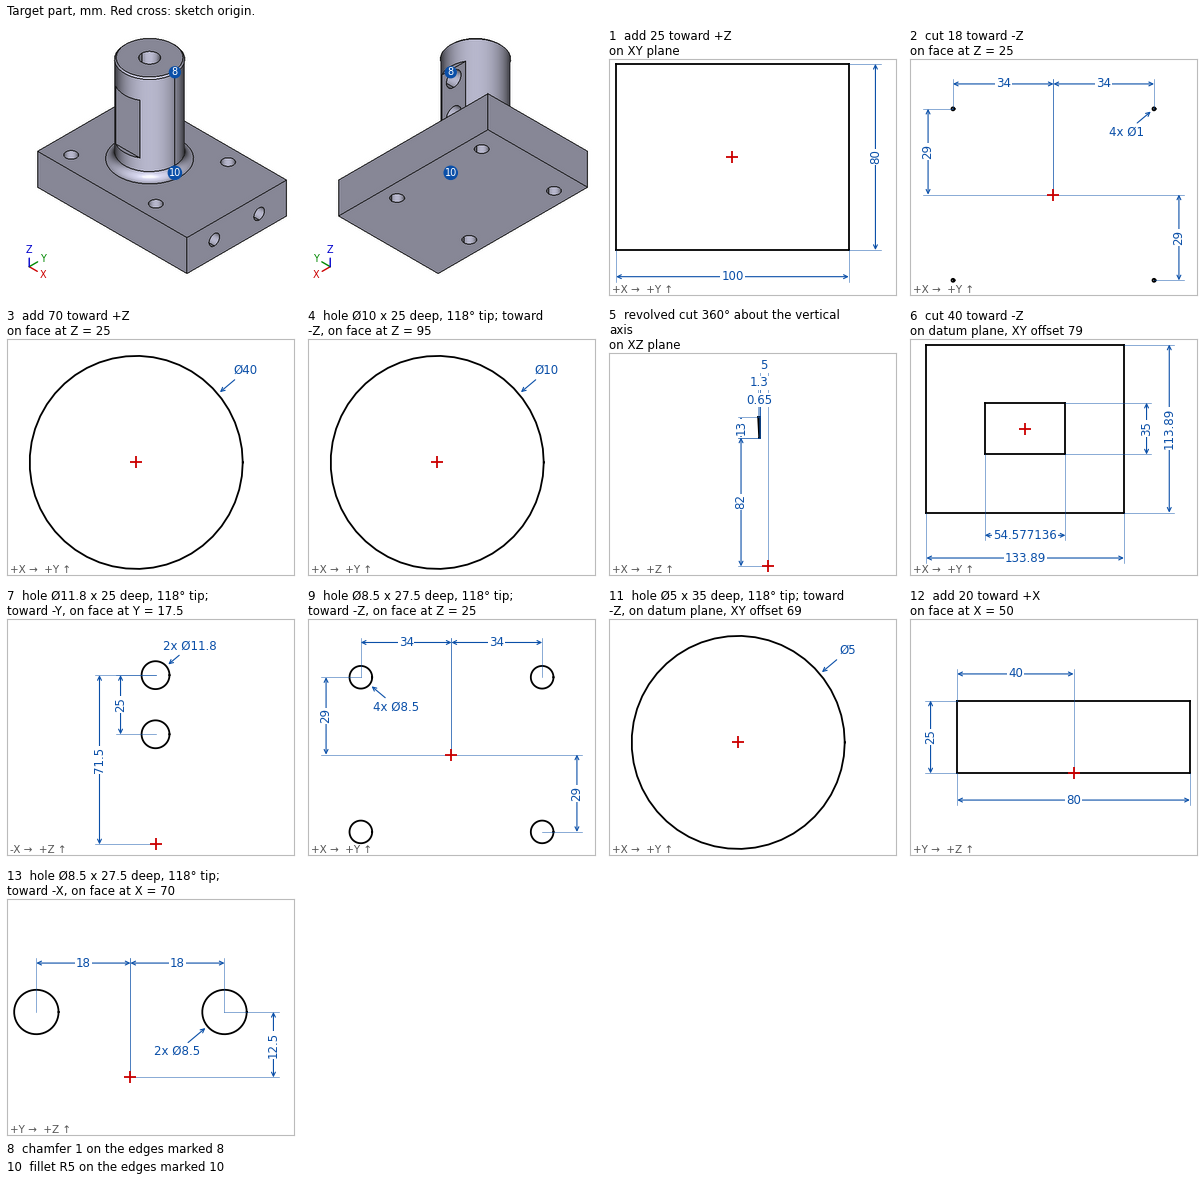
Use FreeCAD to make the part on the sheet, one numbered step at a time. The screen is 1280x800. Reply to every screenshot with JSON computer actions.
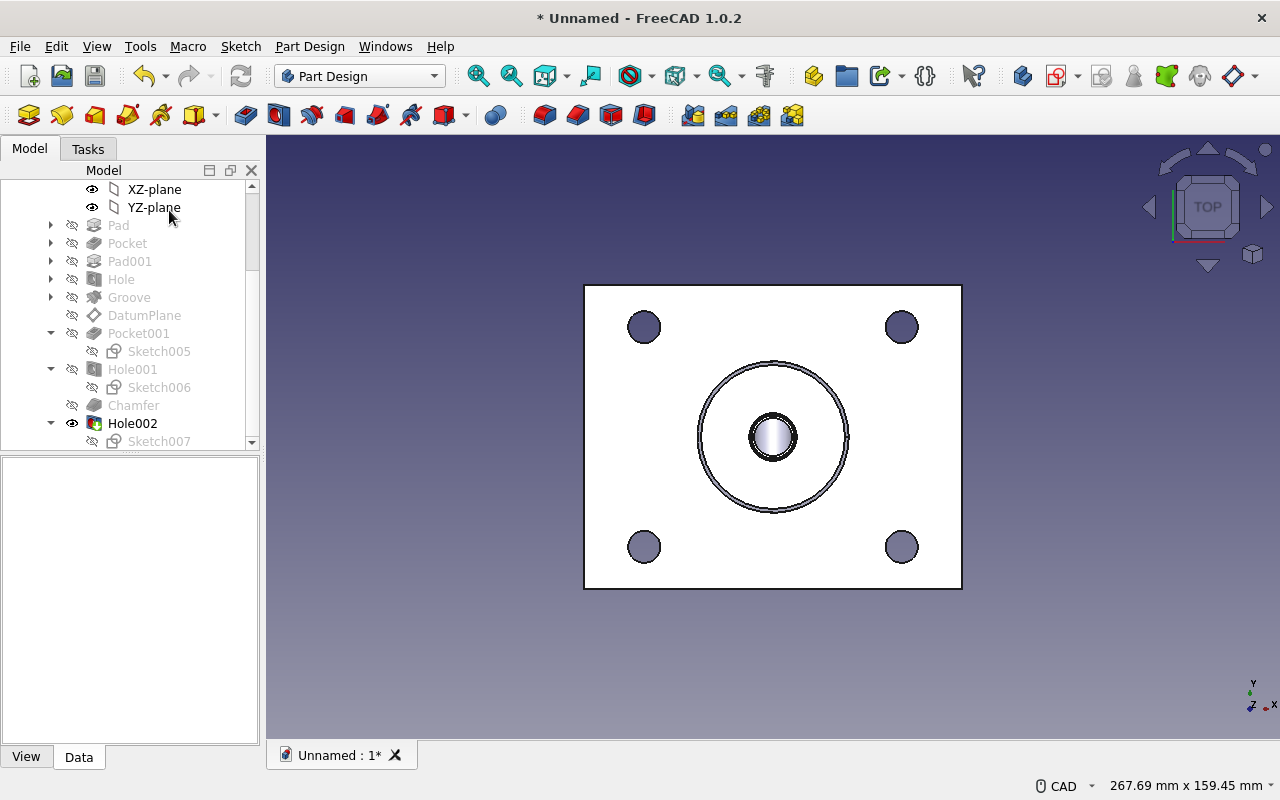
{"action": "key", "text": "0"}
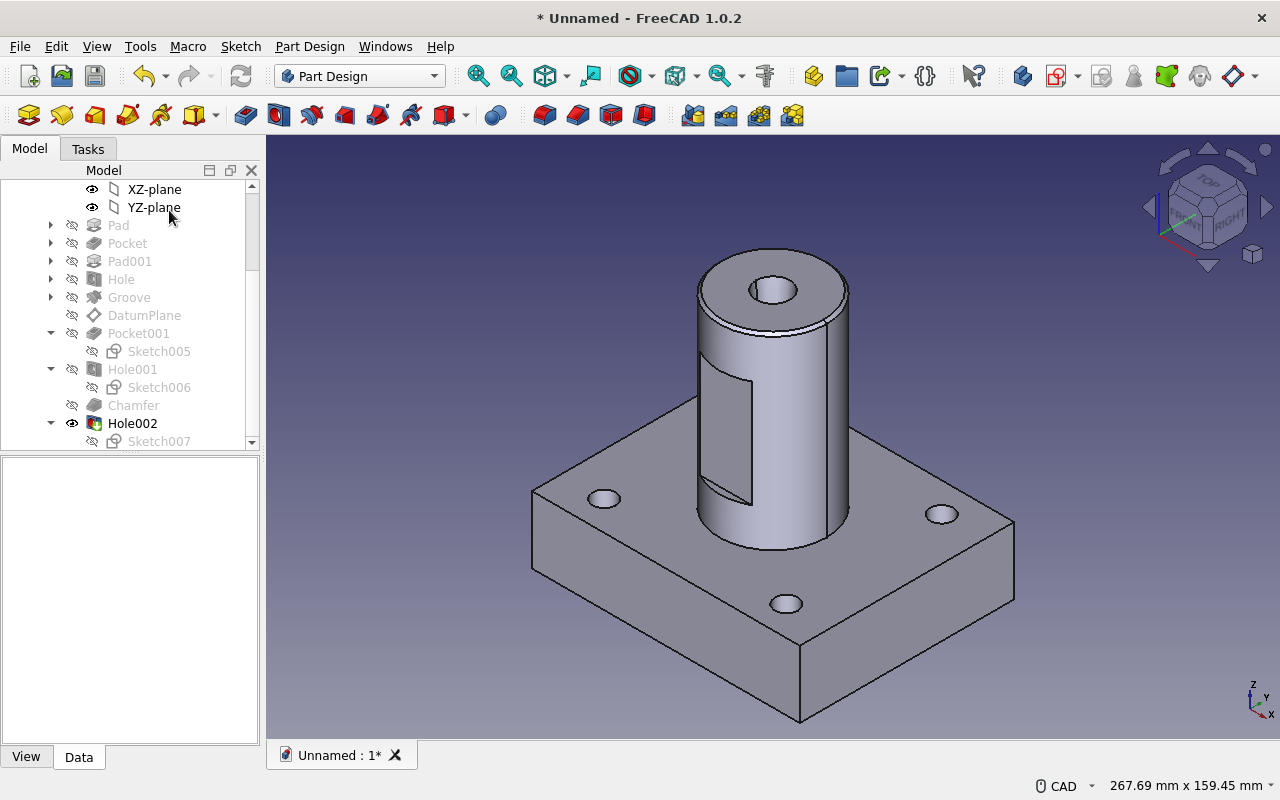
{"action": "key", "text": "1"}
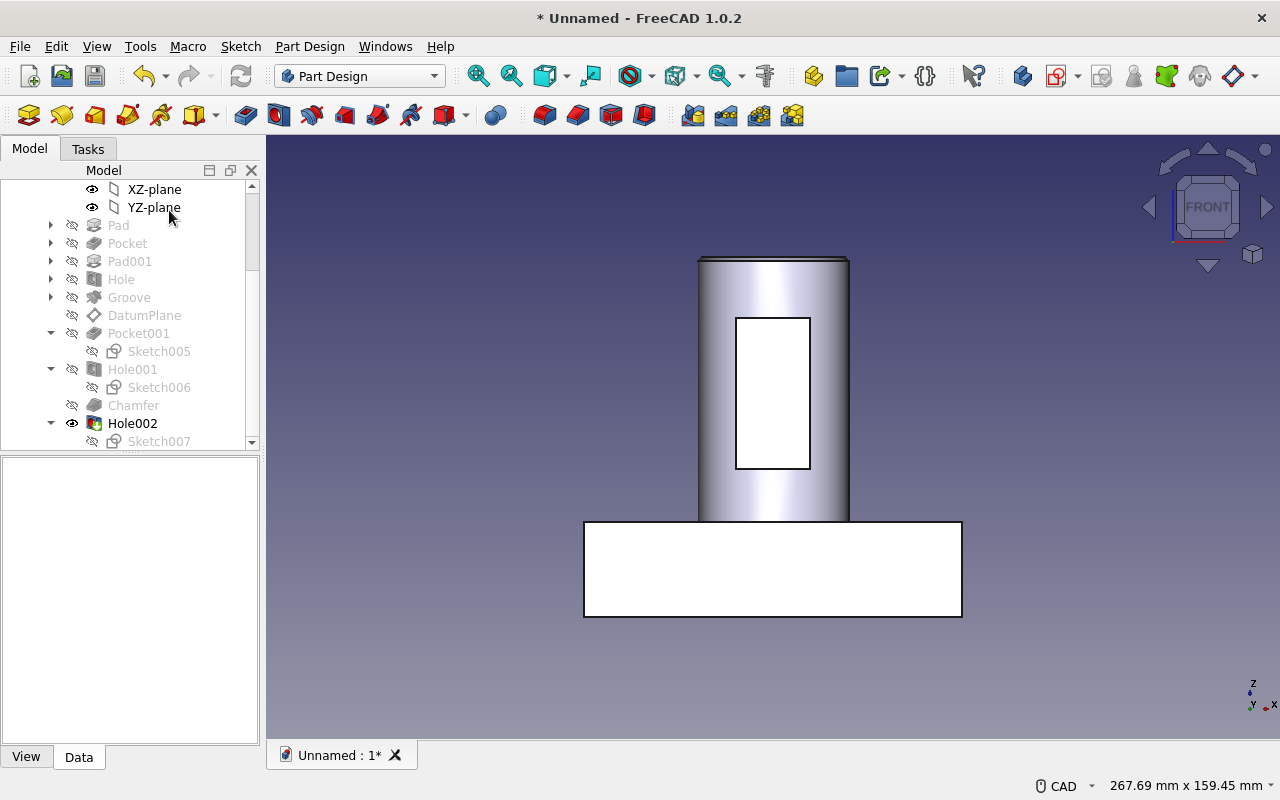
{"action": "key", "text": "3"}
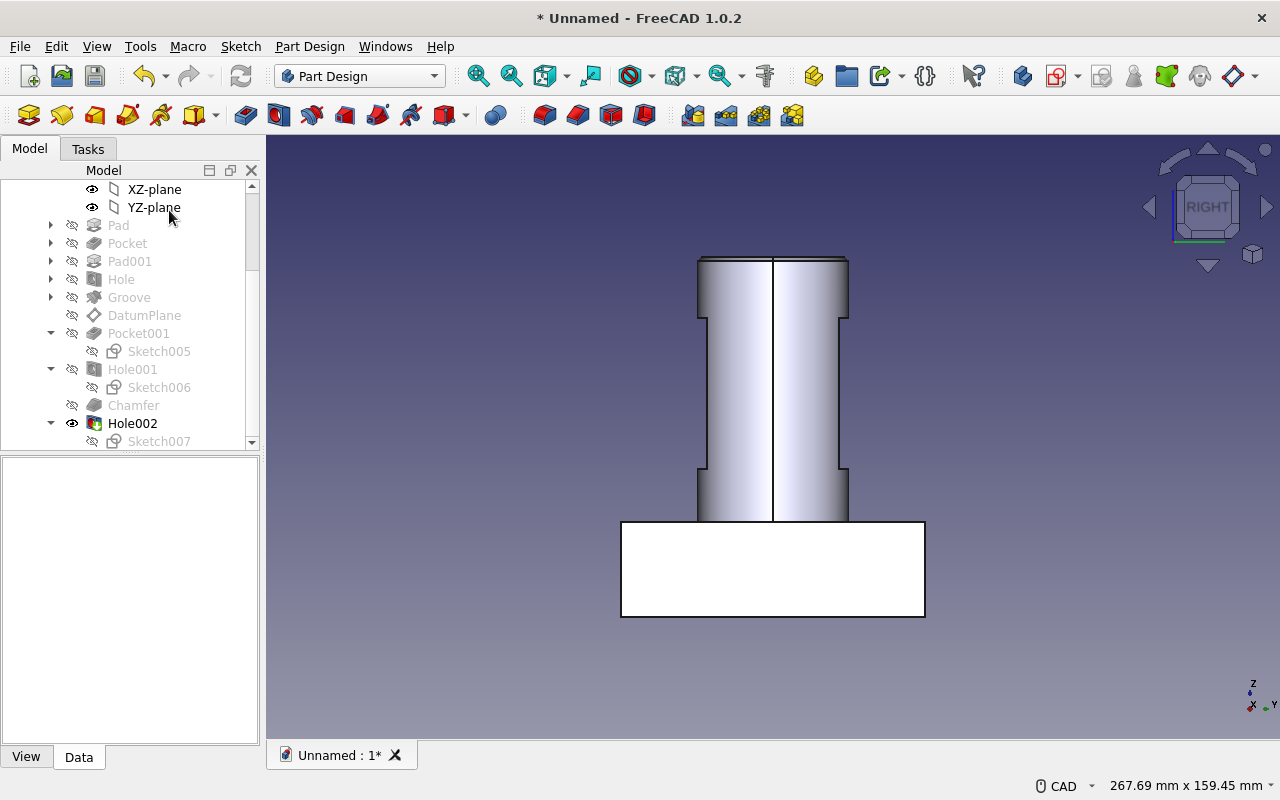
{"action": "key", "text": "5"}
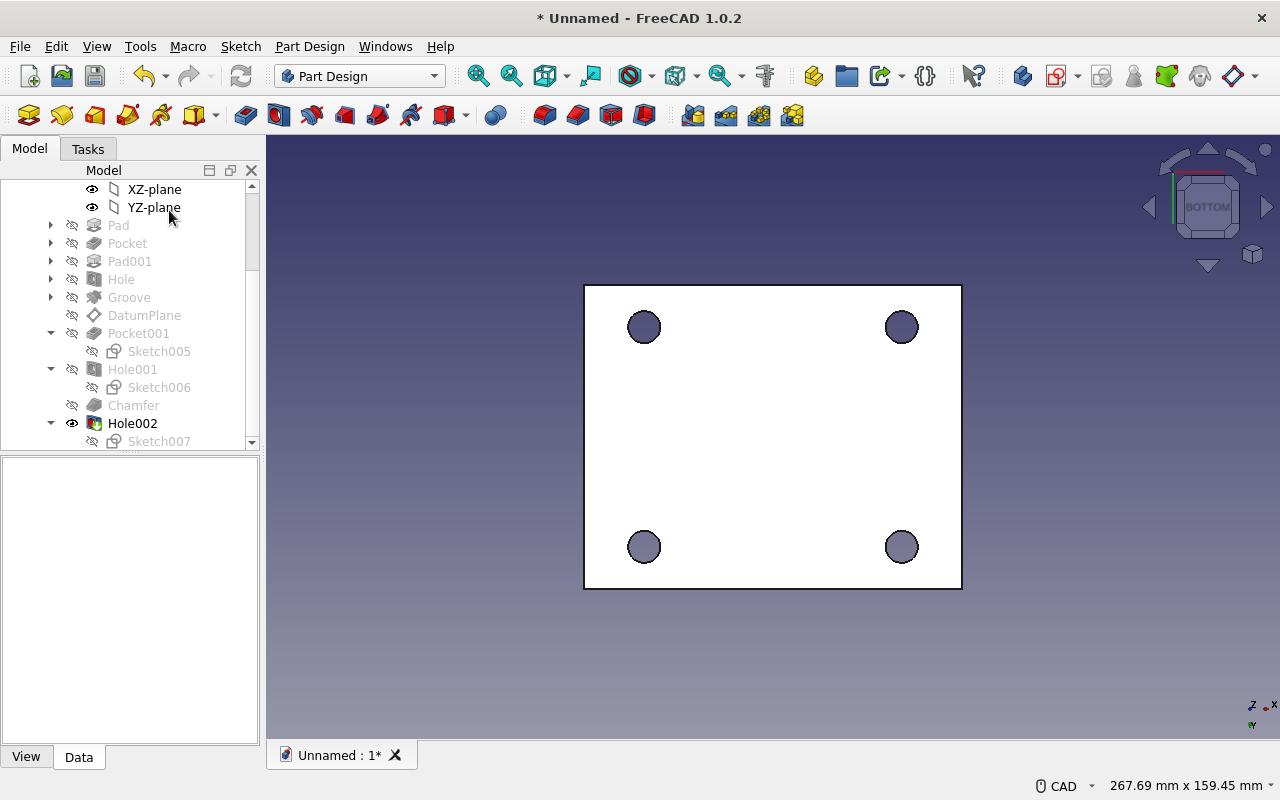
{"action": "key", "text": "4"}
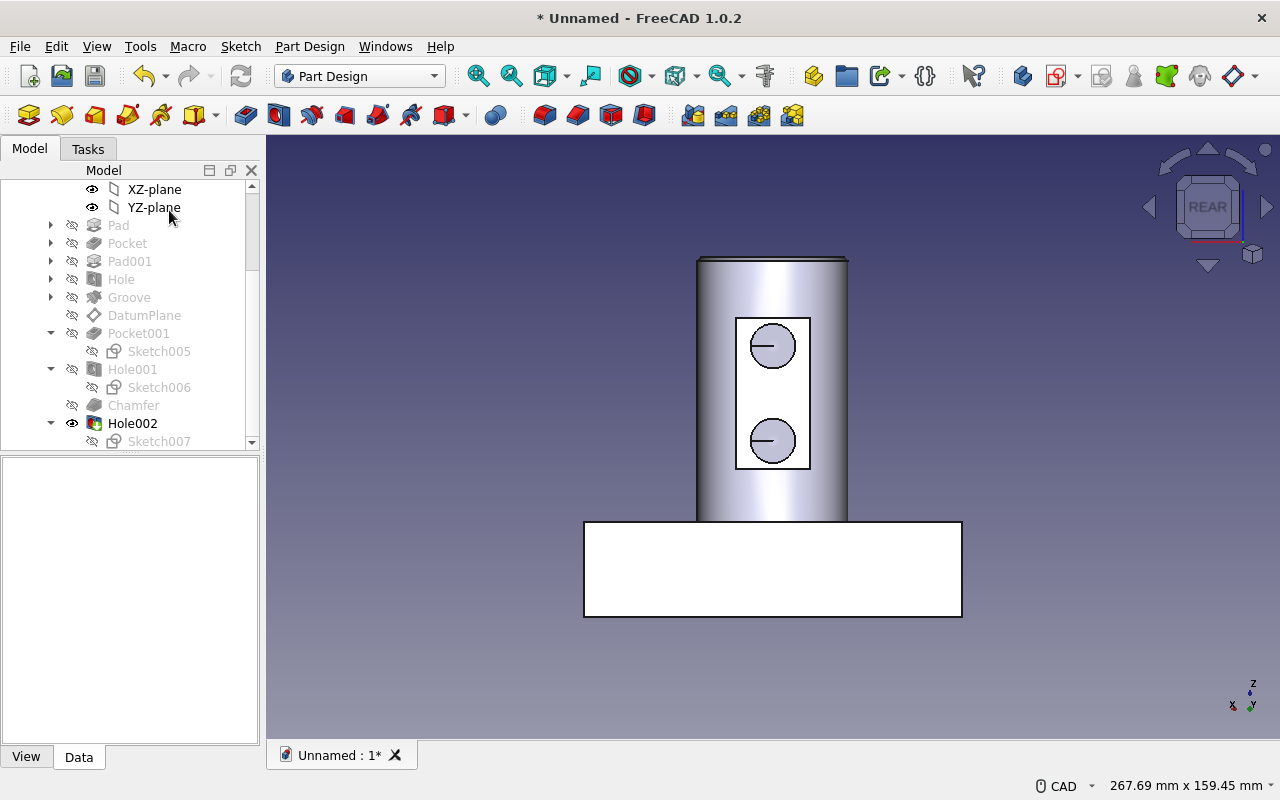
{"action": "key", "text": "6"}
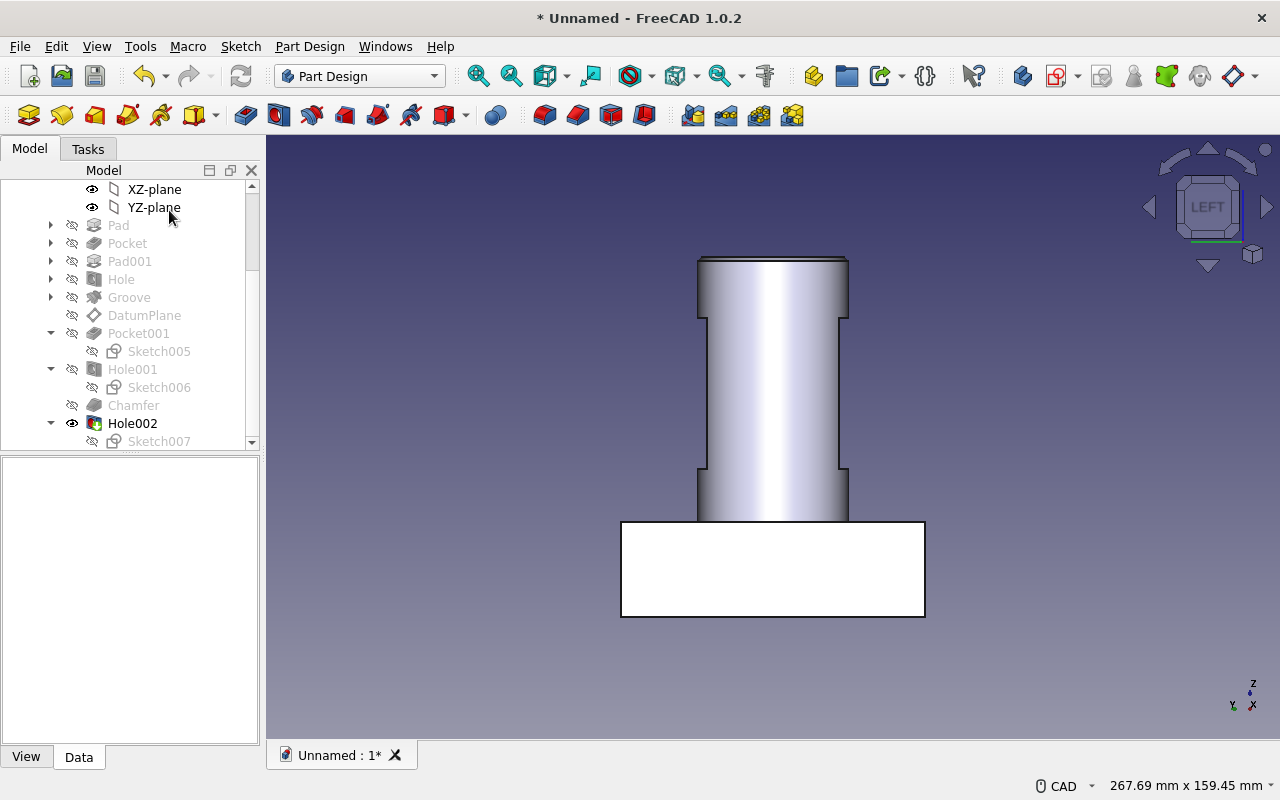
{"action": "key", "text": "v 3"}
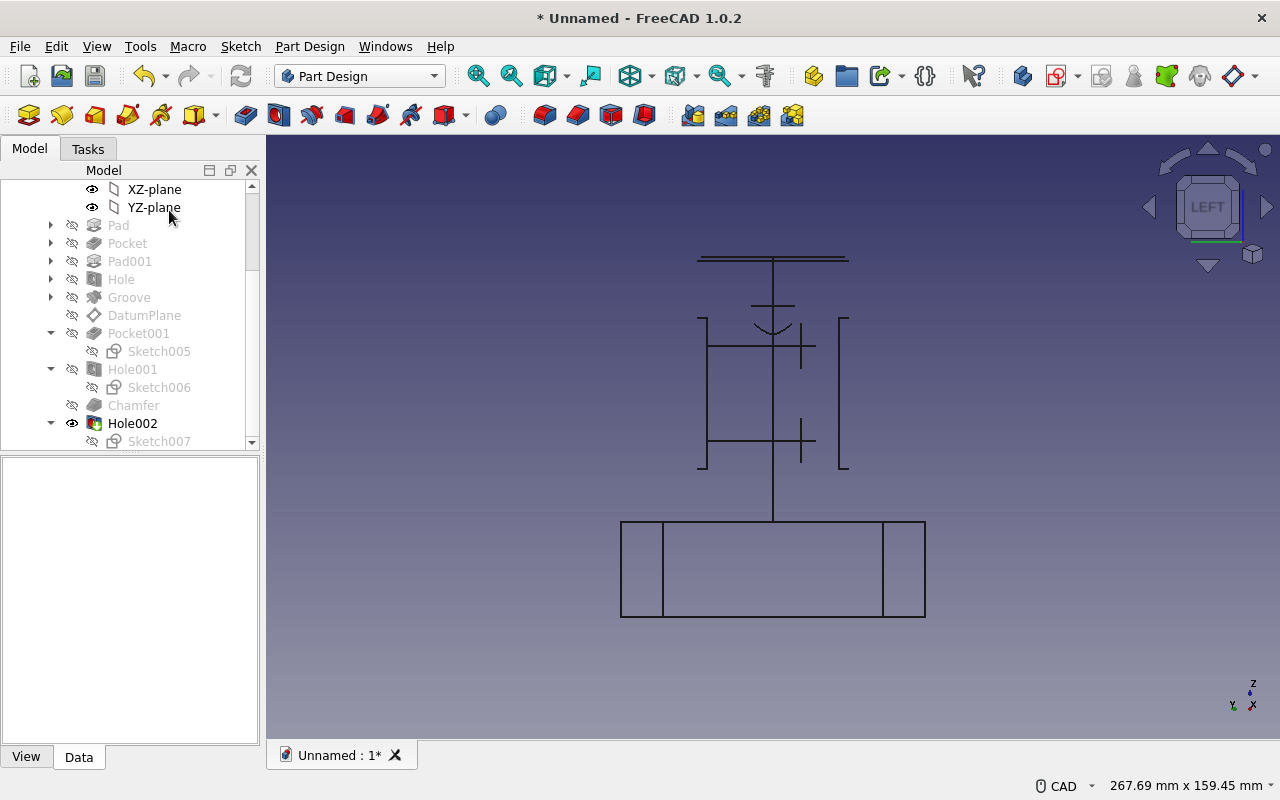
{"action": "key", "text": "0"}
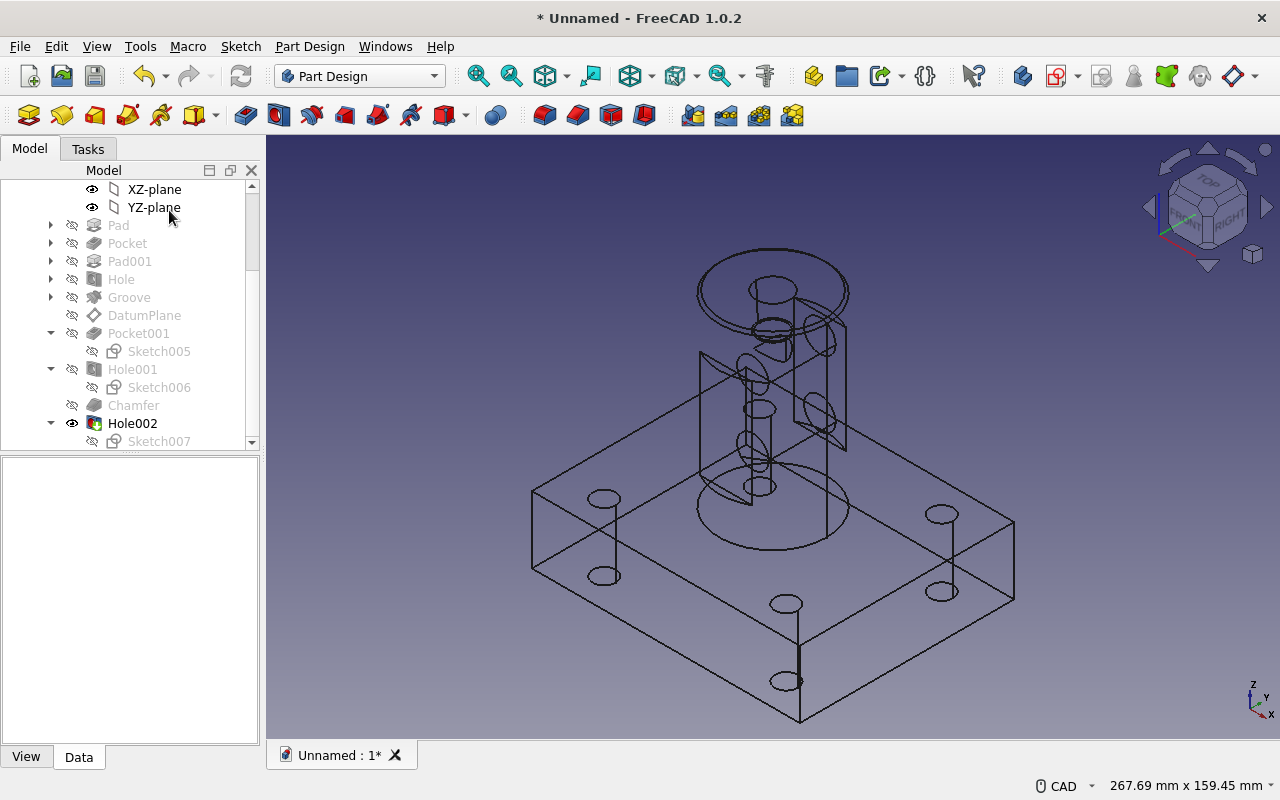
{"action": "left_click", "coordinate": [719, 475]}